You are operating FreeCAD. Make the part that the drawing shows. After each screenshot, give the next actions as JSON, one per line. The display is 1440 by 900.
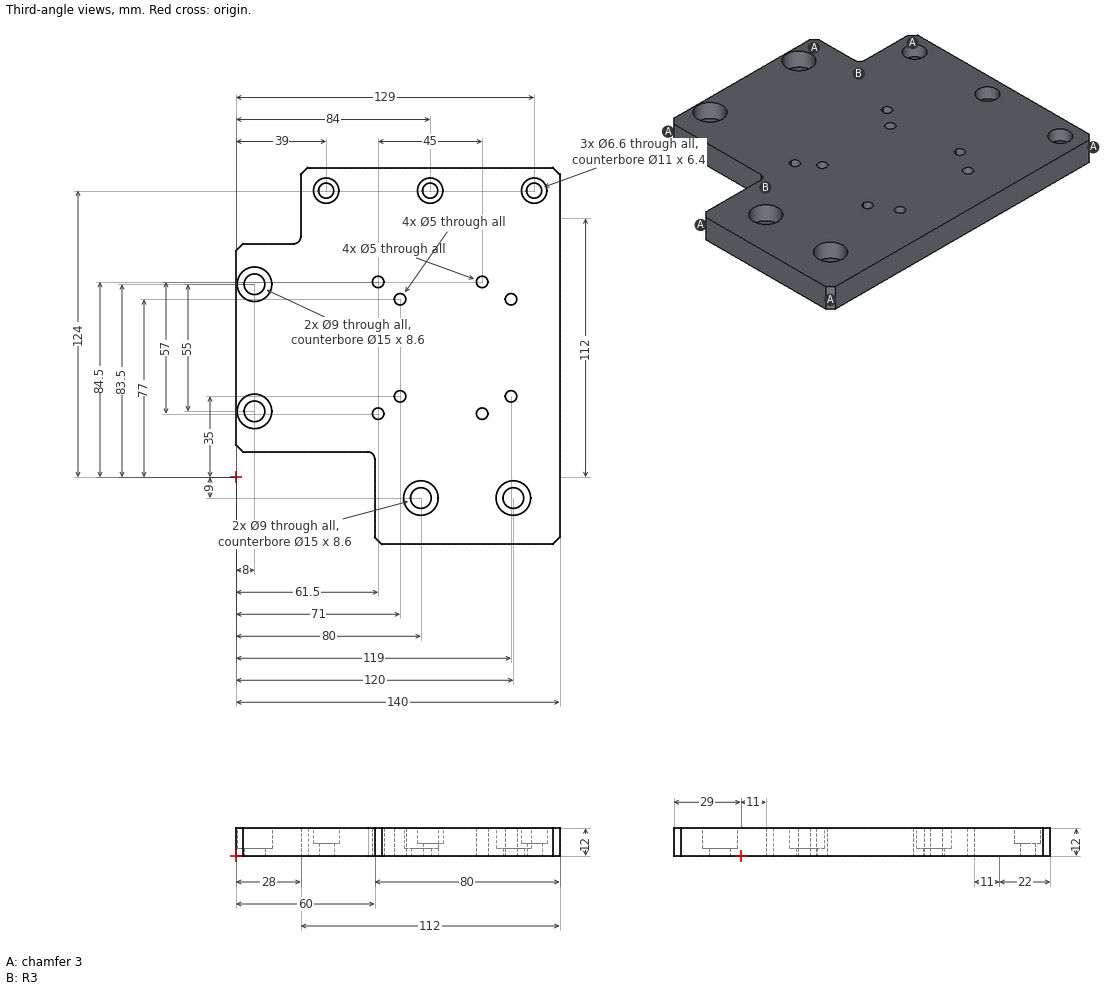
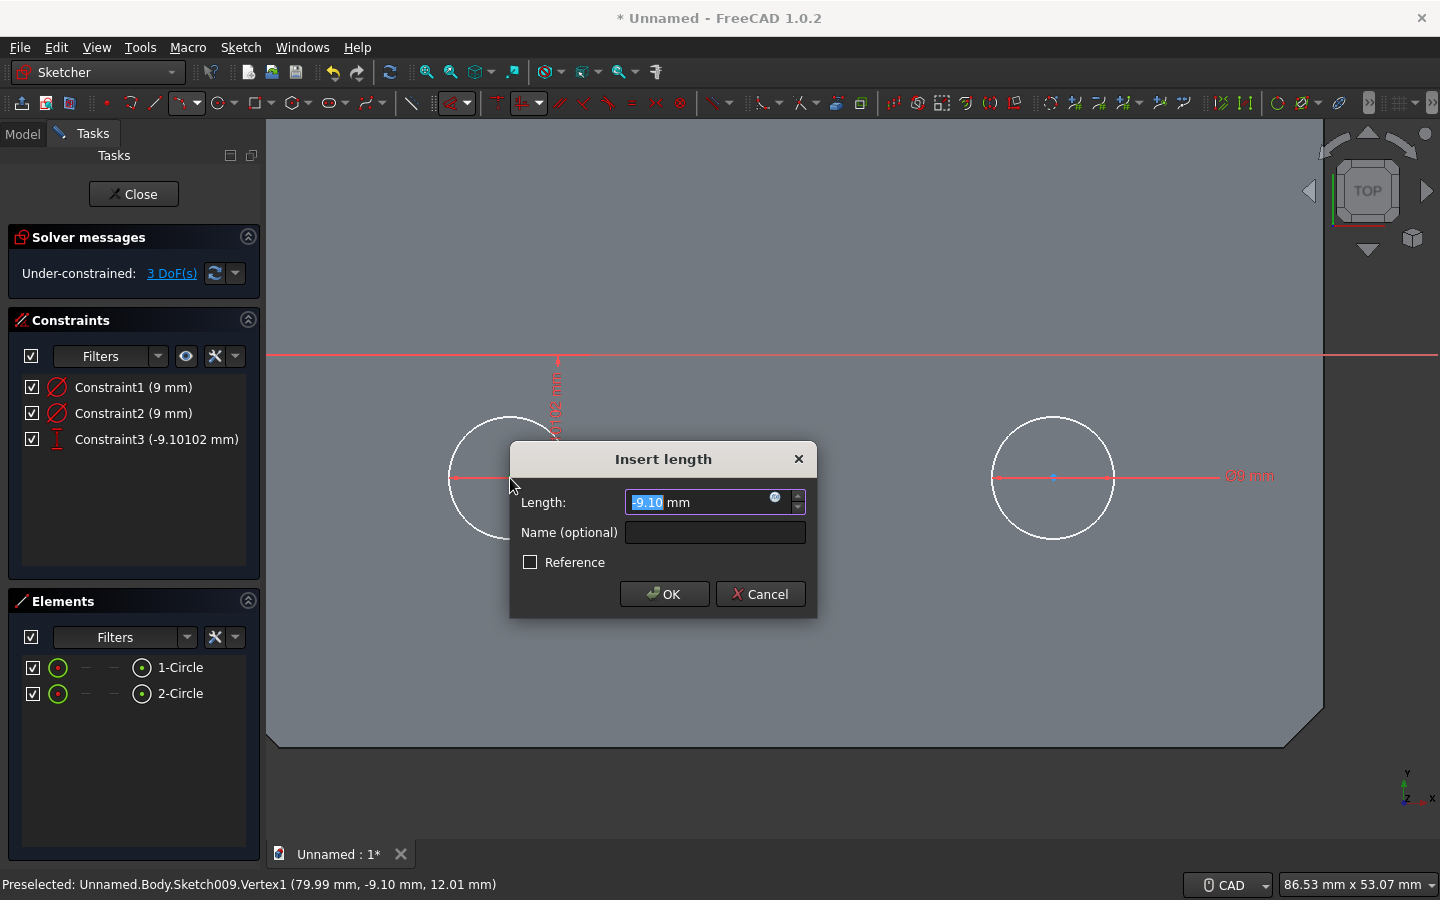
{"action": "type", "text": "-9"}
{"action": "key", "text": "Return"}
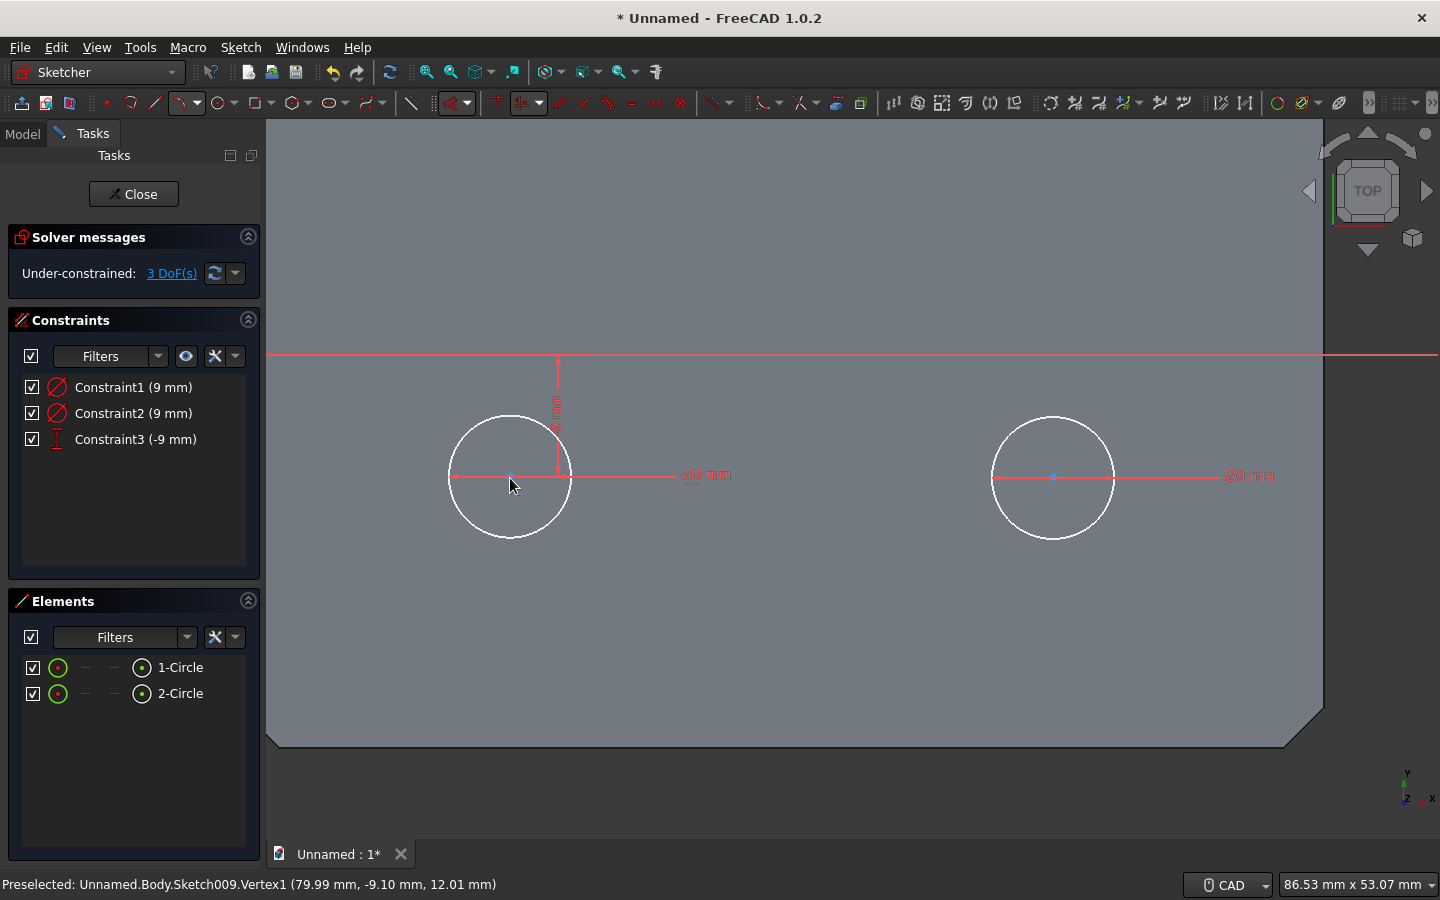
{"action": "left_click", "coordinate": [1053, 478]}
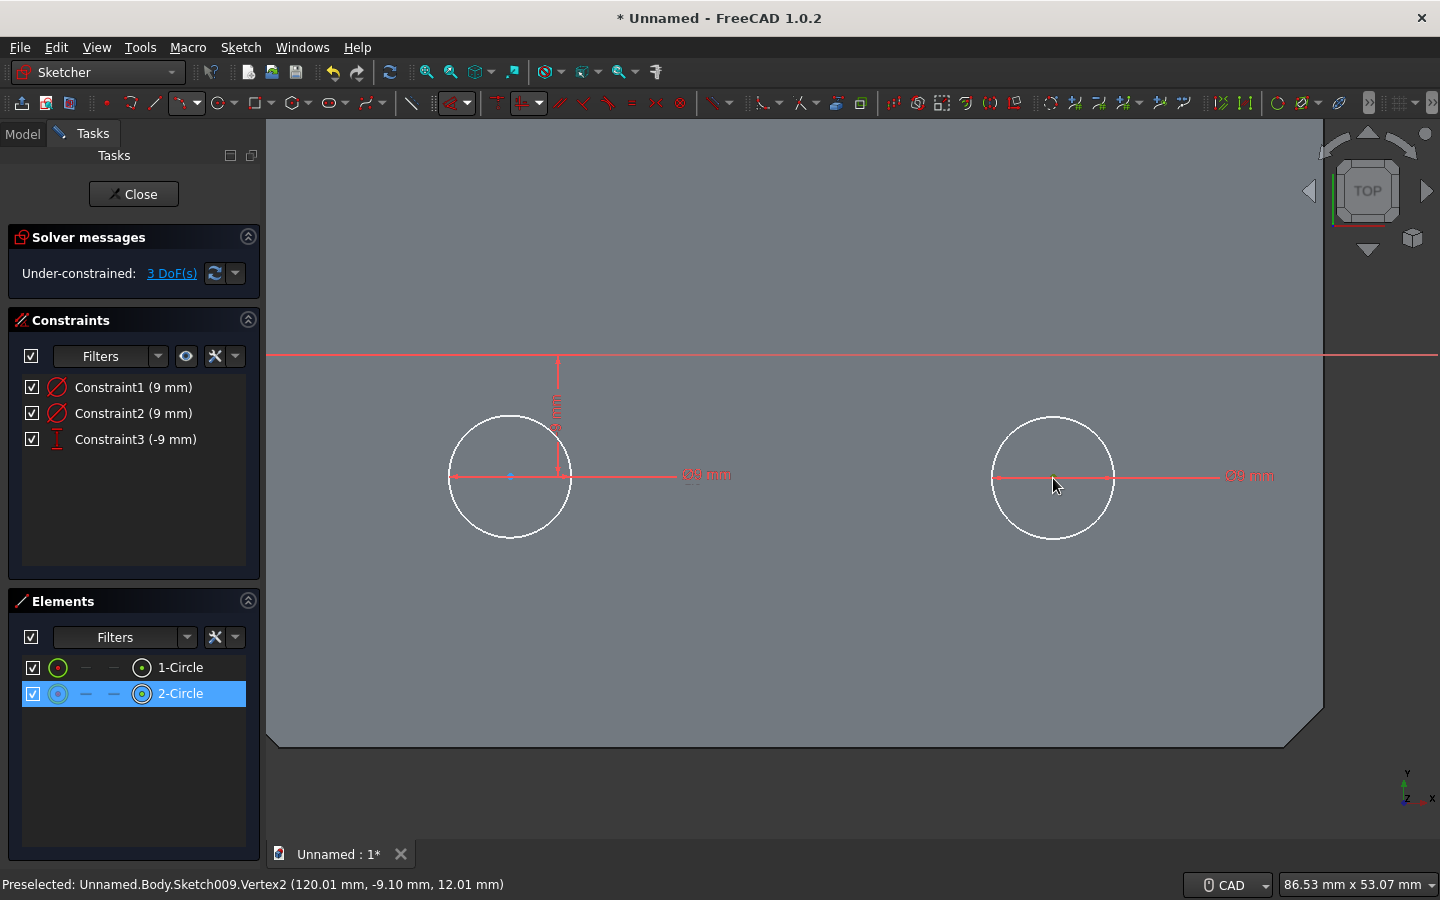
{"action": "key", "text": "i"}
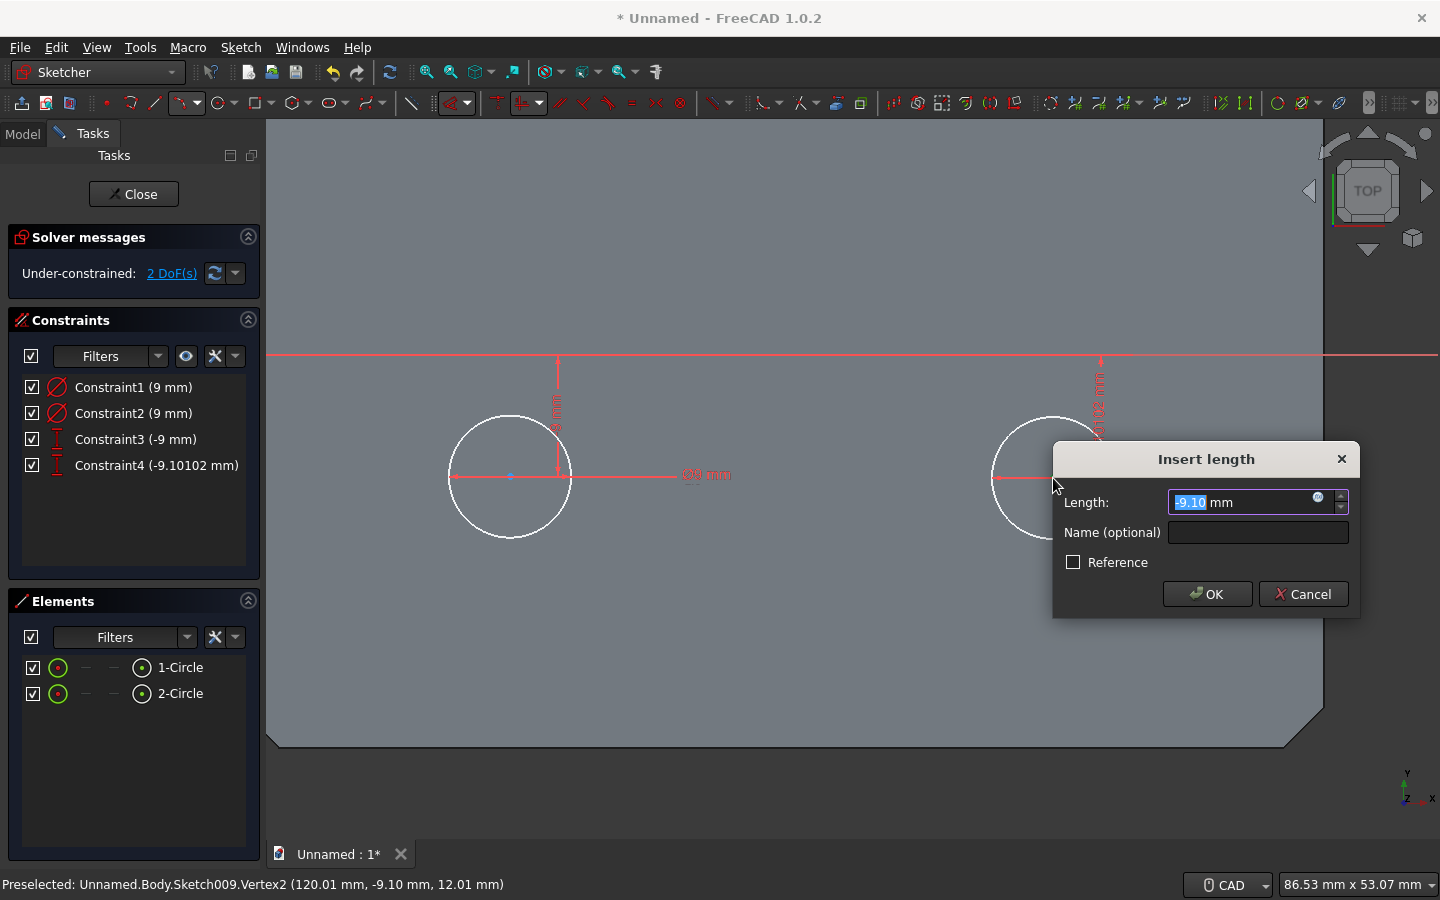
{"action": "type", "text": "-9"}
{"action": "key", "text": "Return"}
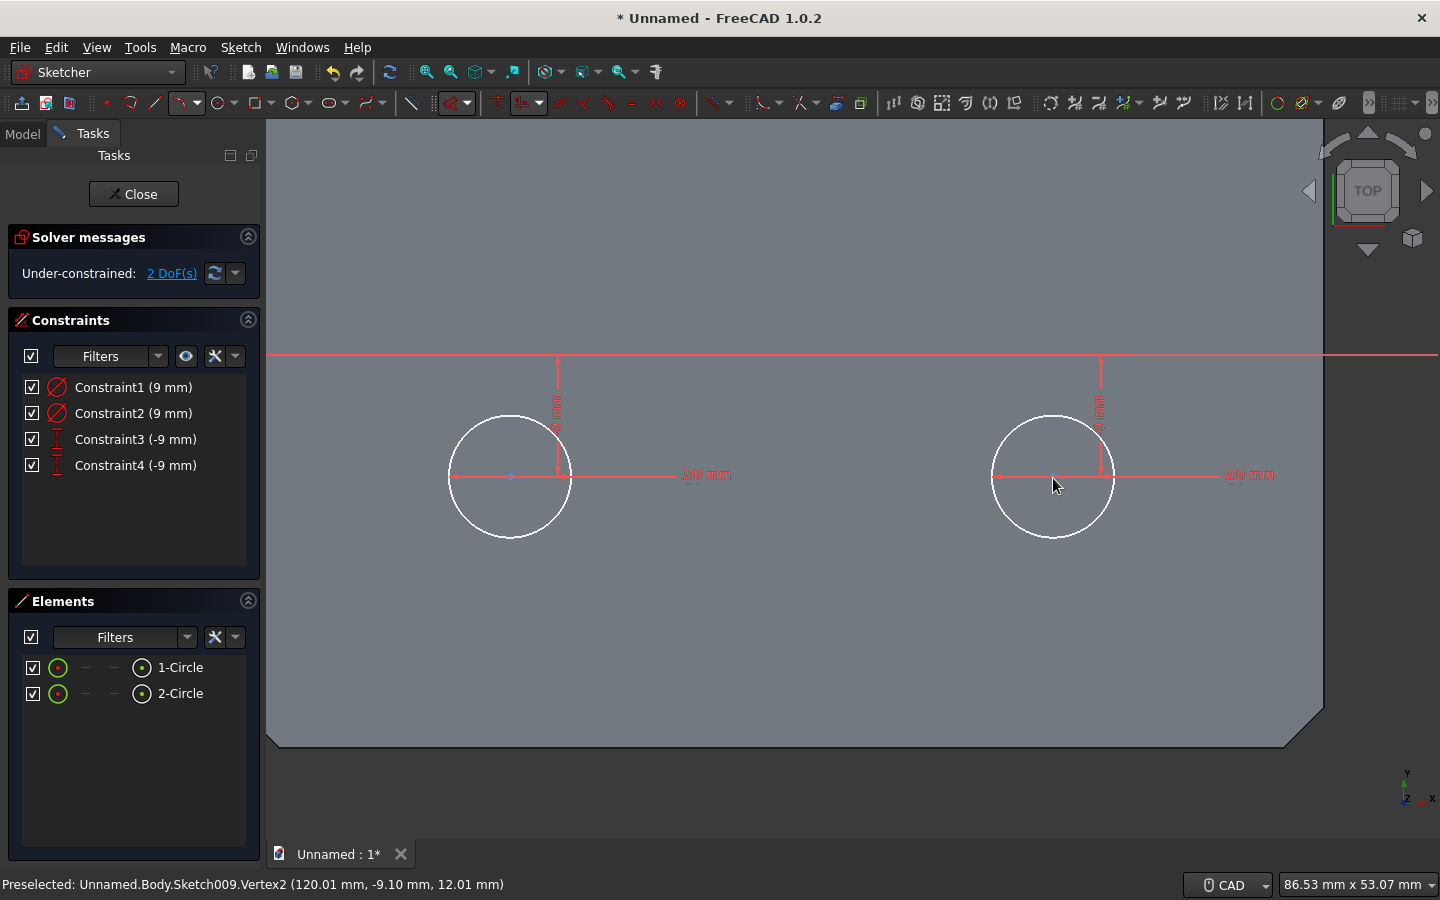
{"action": "left_click", "coordinate": [510, 477]}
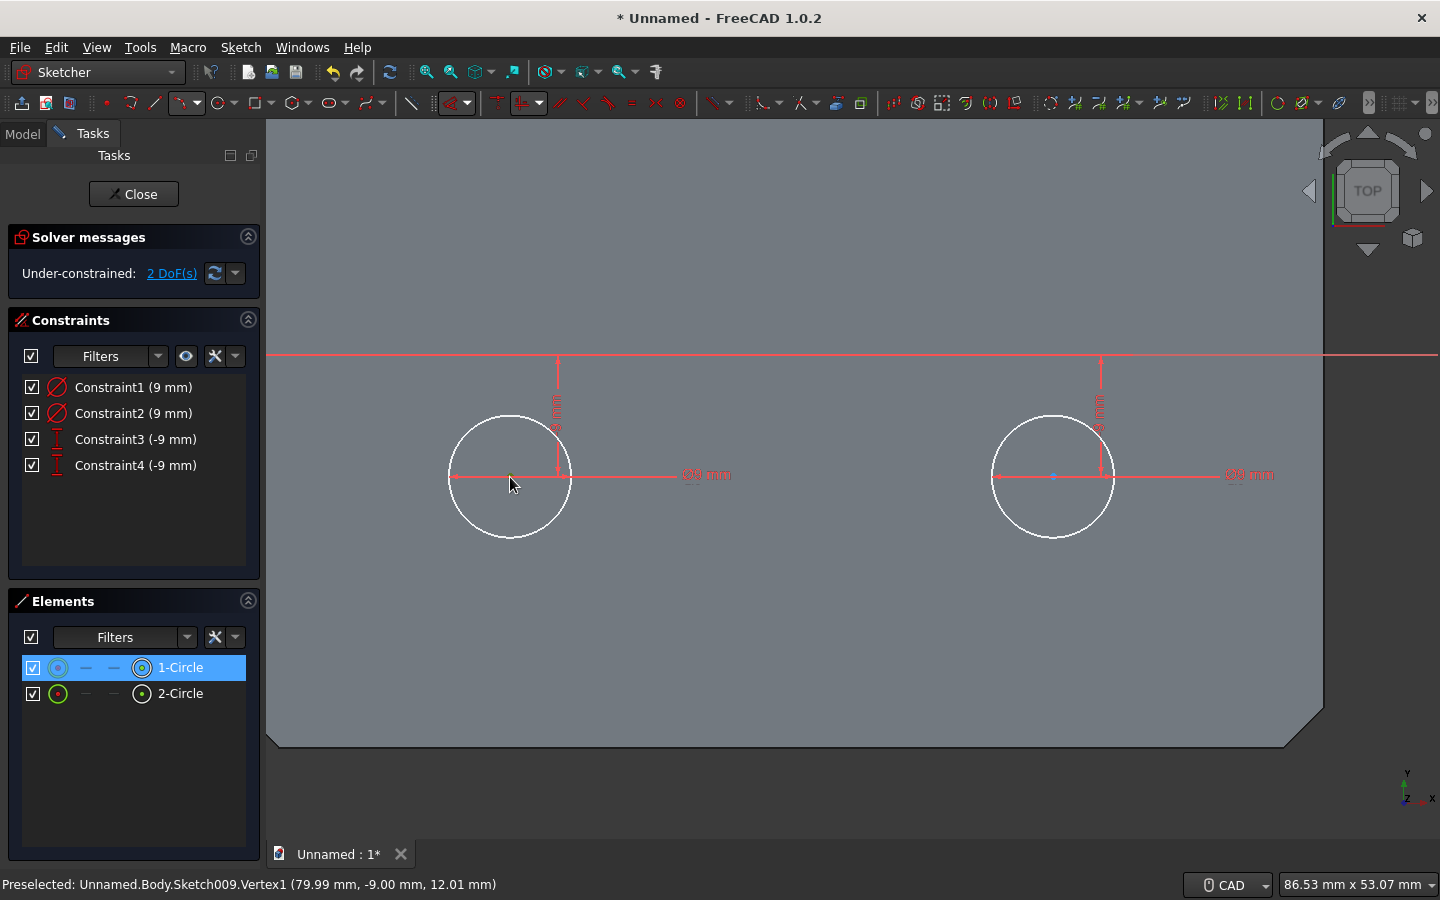
{"action": "left_click", "coordinate": [470, 104]}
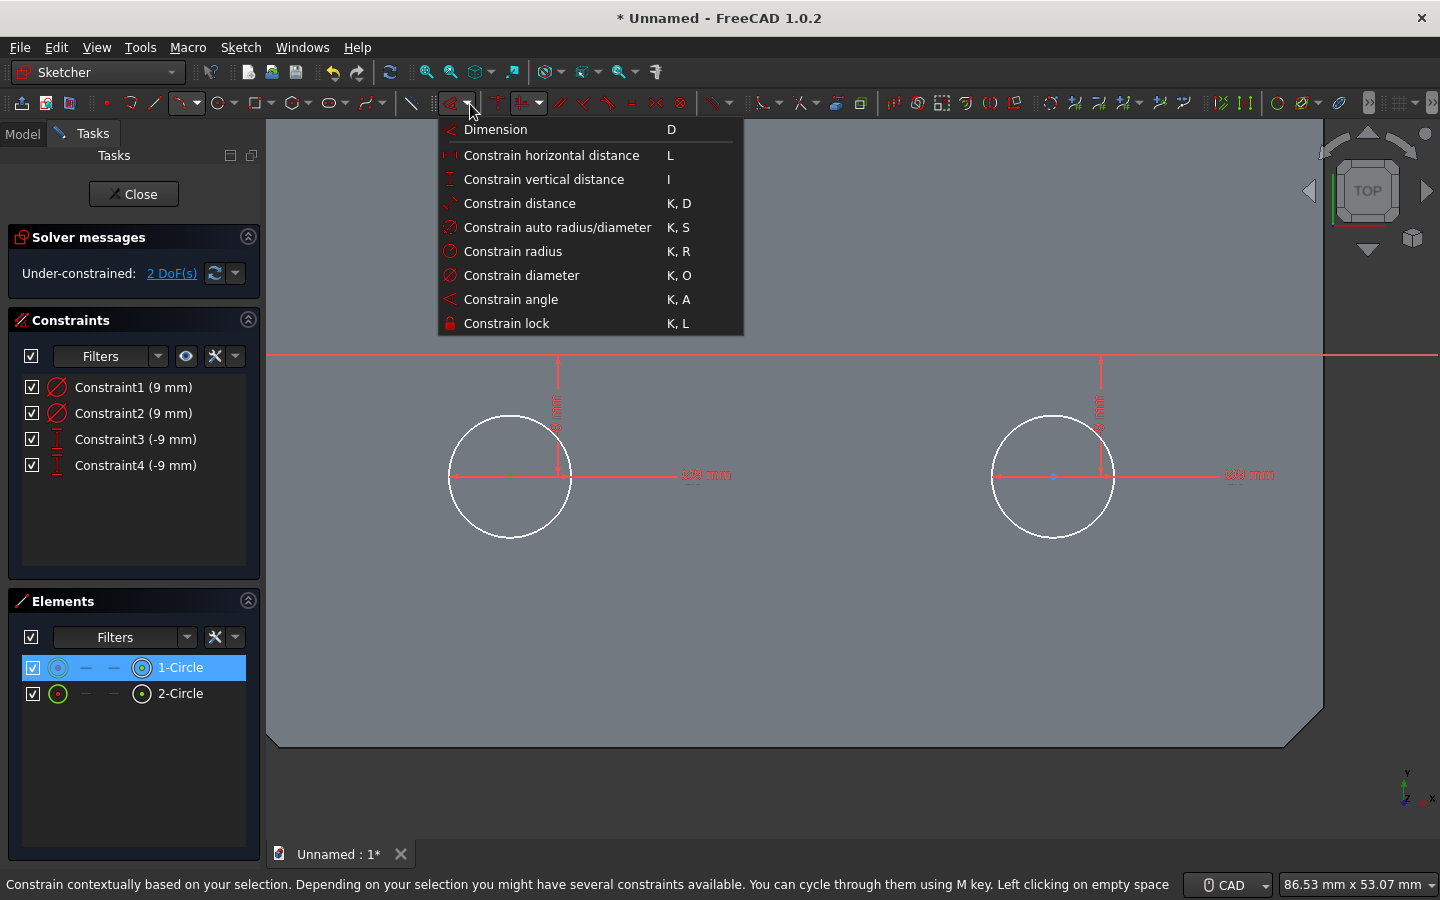
{"action": "left_click", "coordinate": [591, 155]}